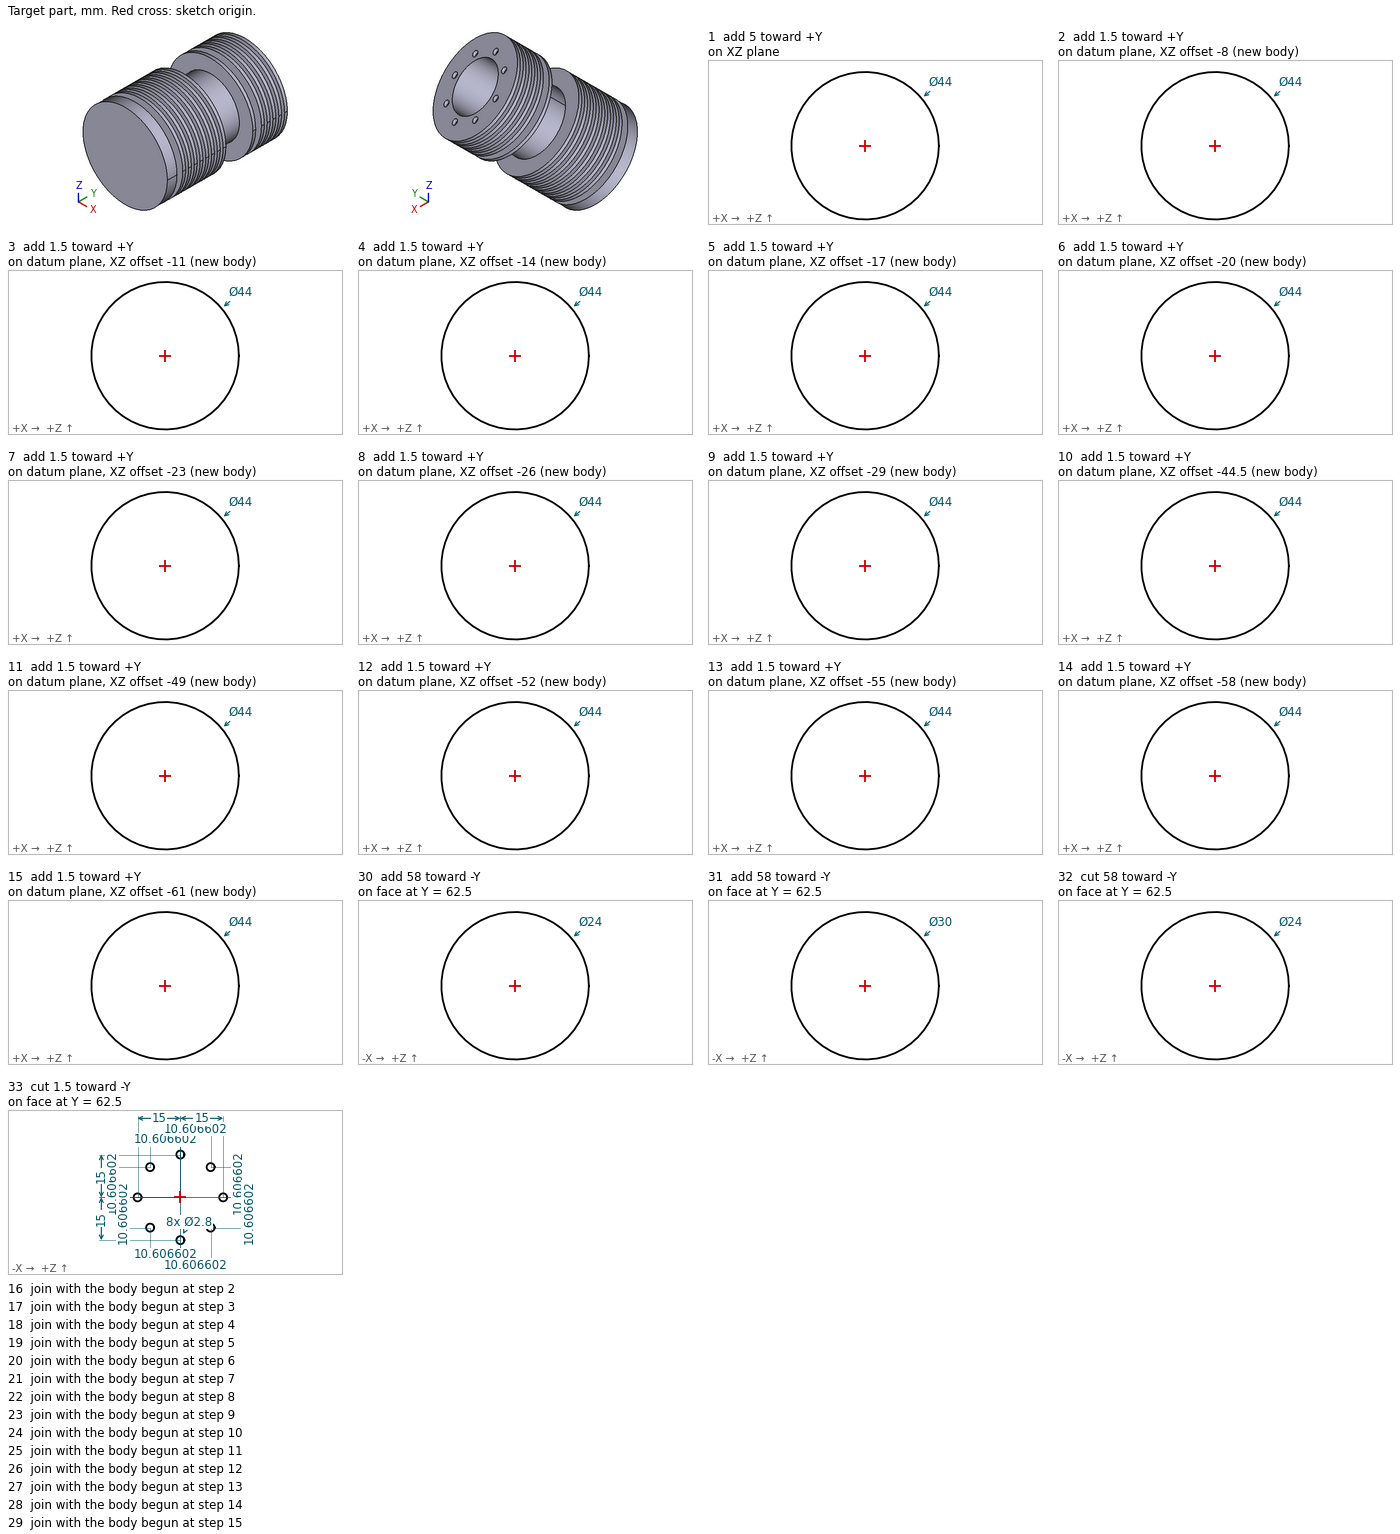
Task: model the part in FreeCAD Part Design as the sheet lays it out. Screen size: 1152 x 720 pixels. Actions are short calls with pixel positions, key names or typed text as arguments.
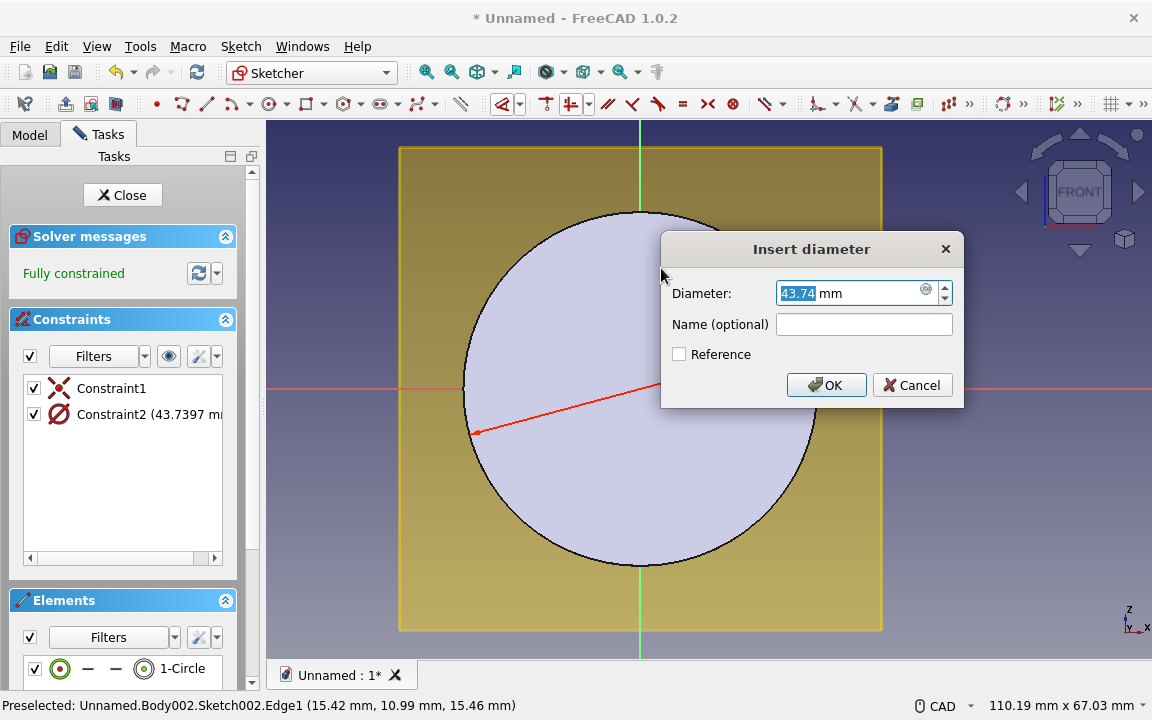
text(44)
key(Return)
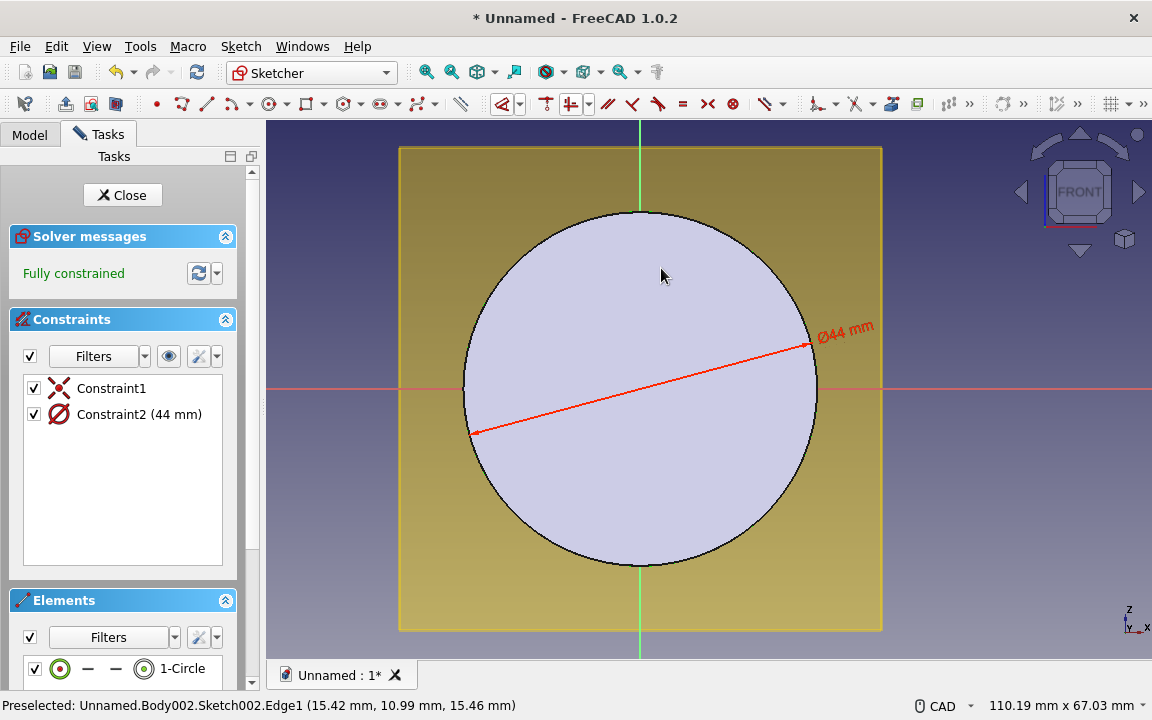
click(123, 195)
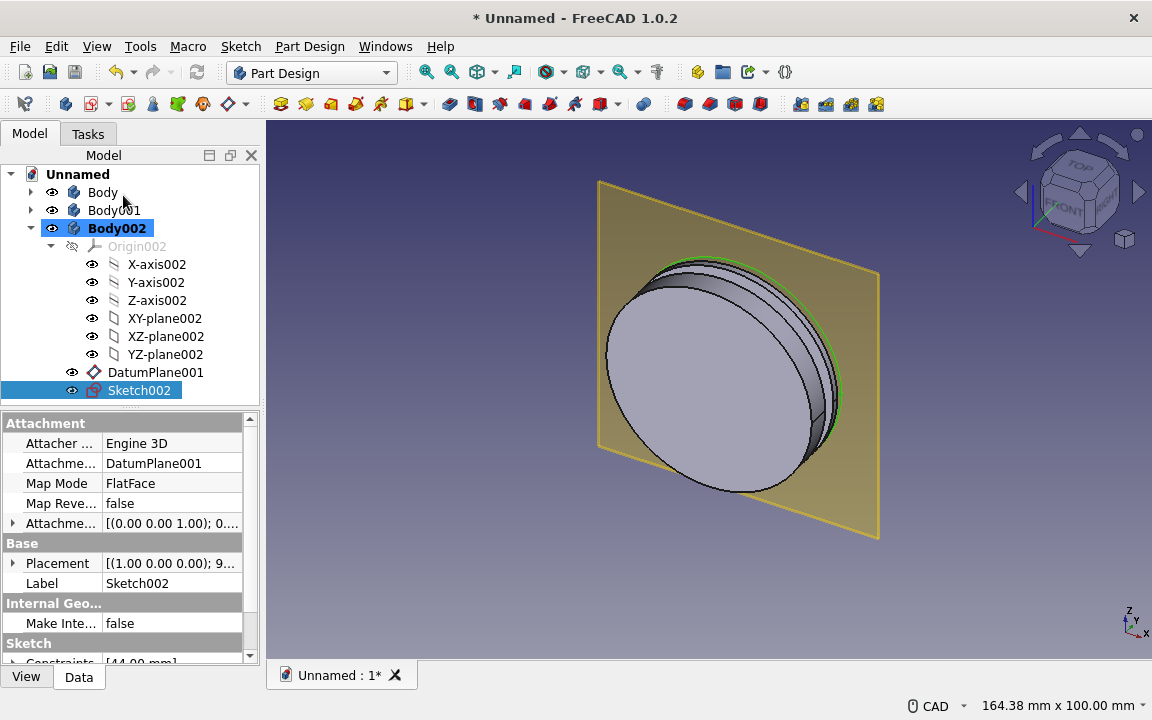
click(281, 104)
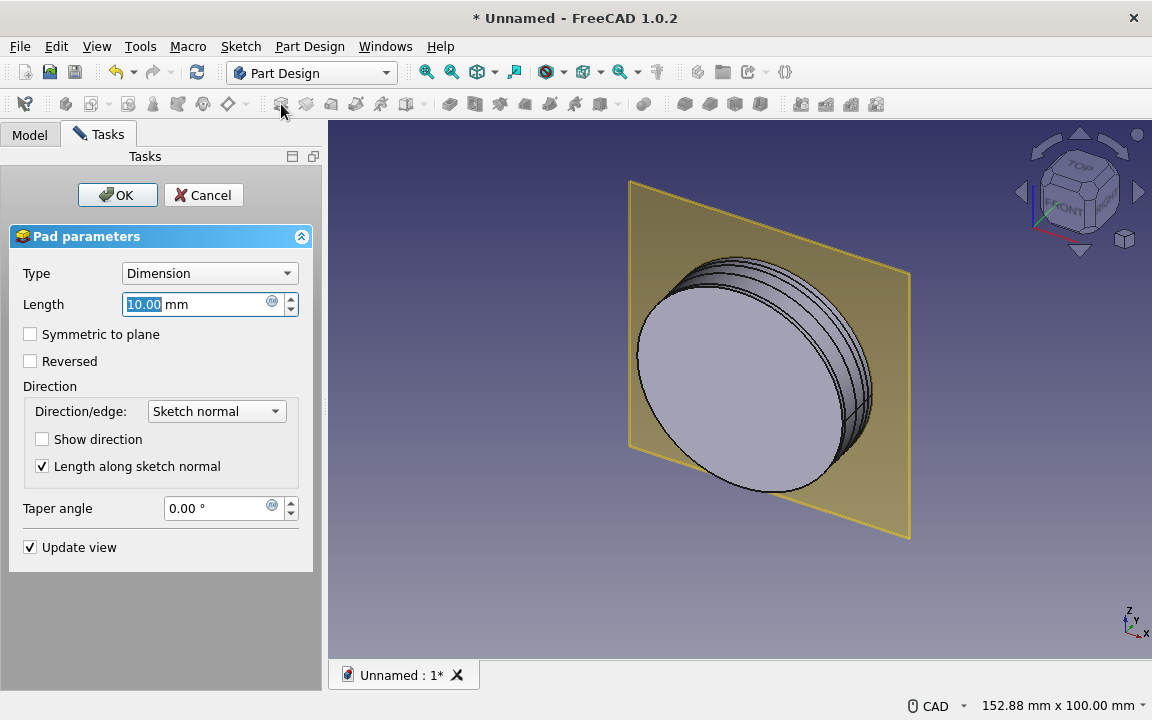
text(1.5)
key(Tab)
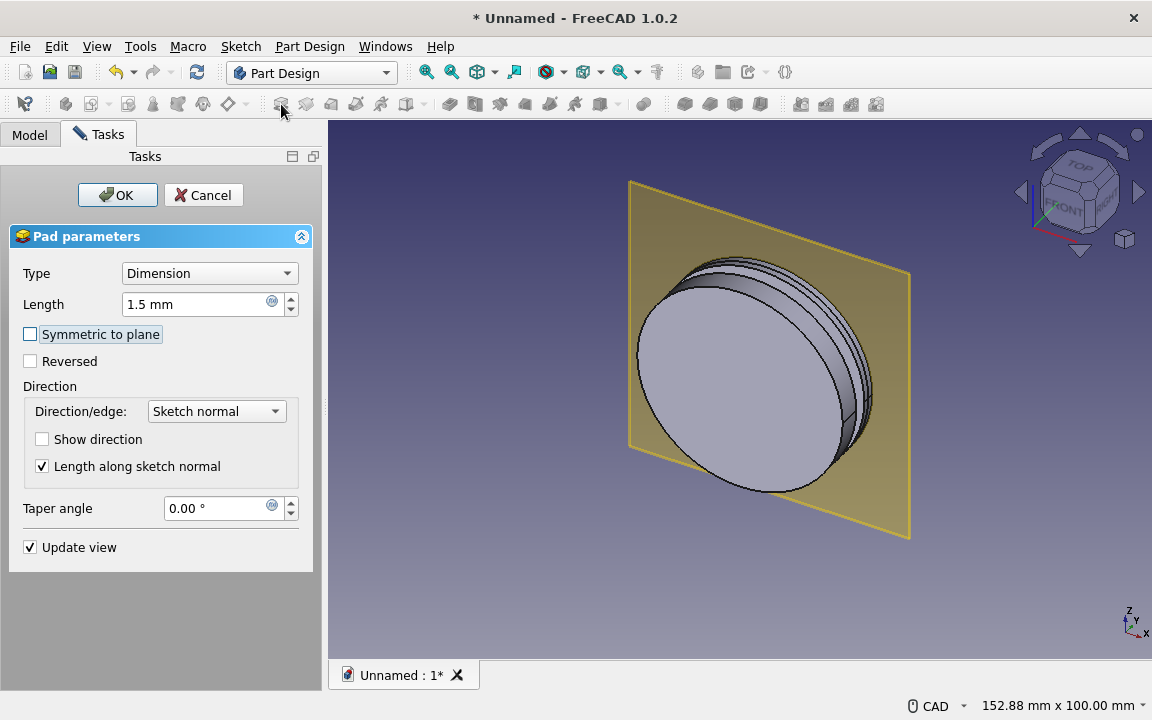
click(31, 361)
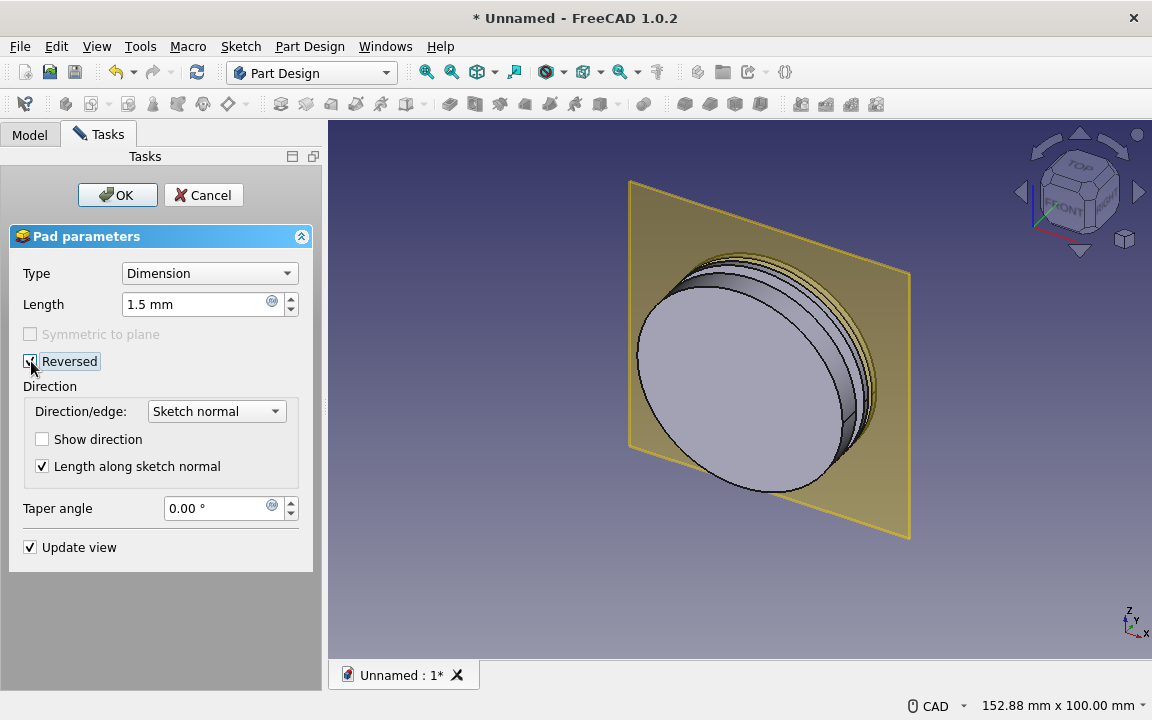
click(118, 195)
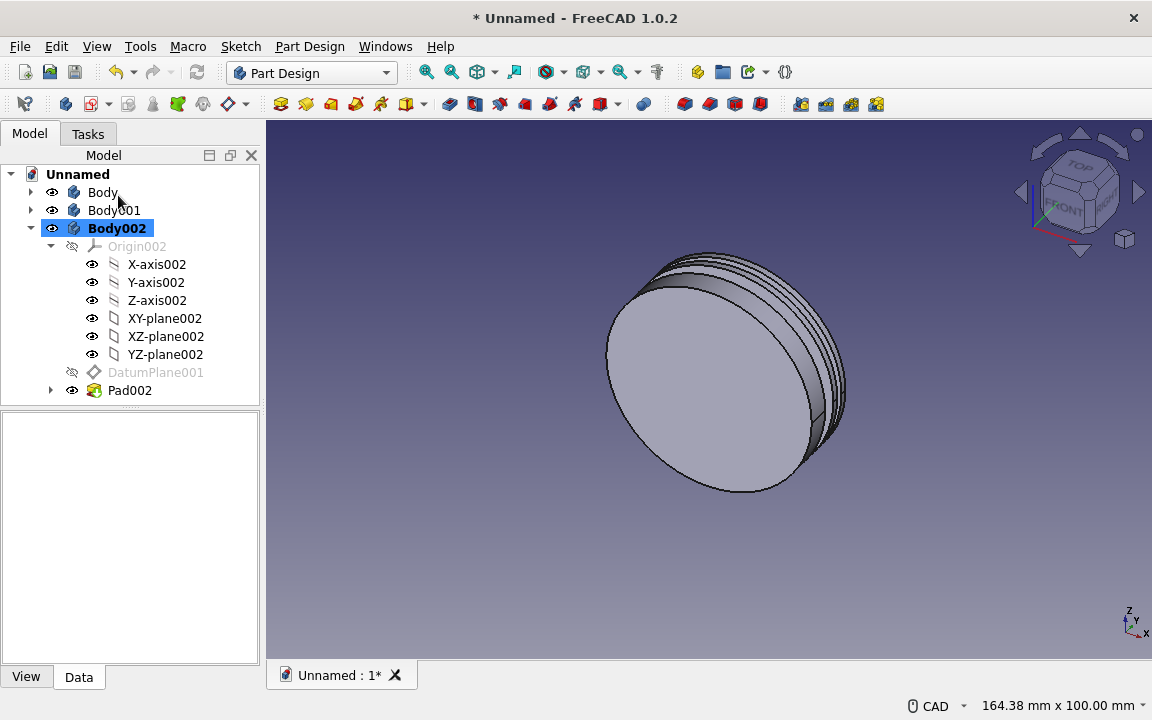
click(66, 104)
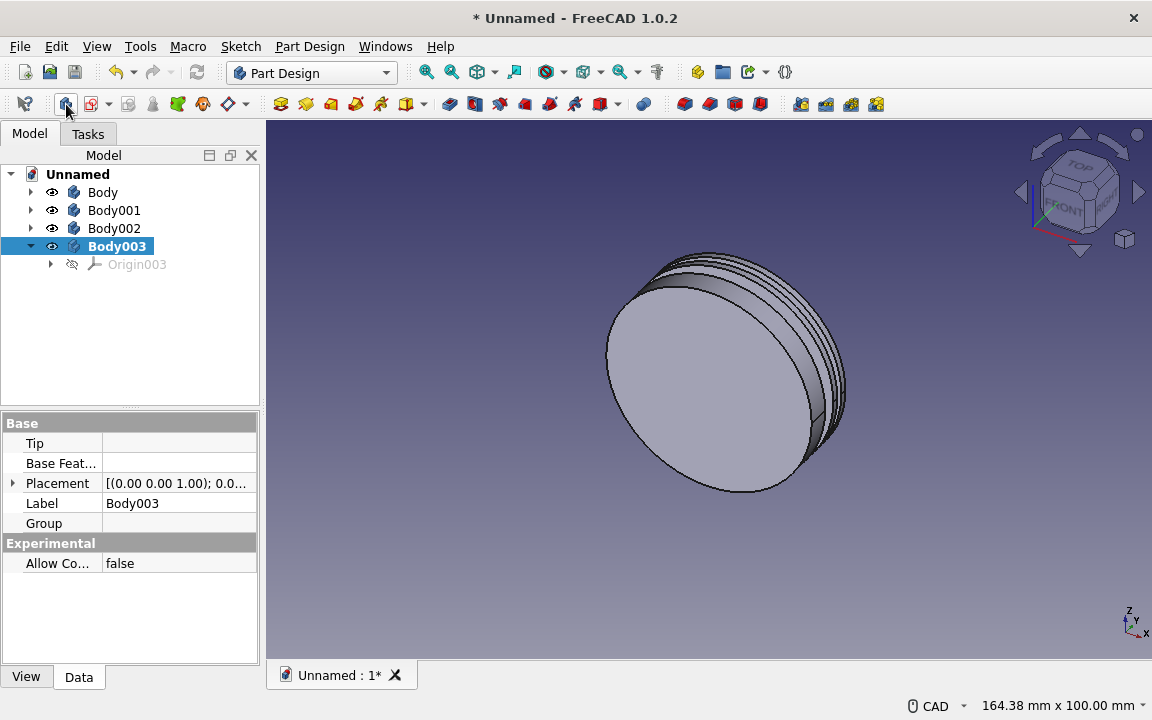
click(51, 264)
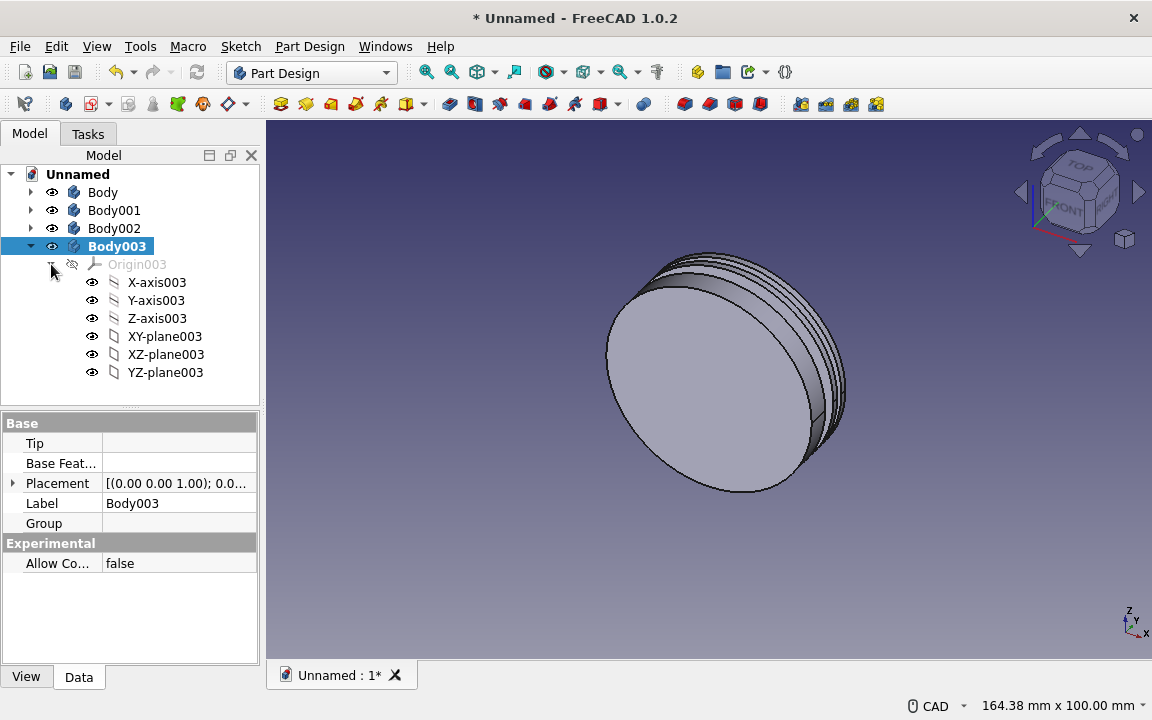
click(137, 354)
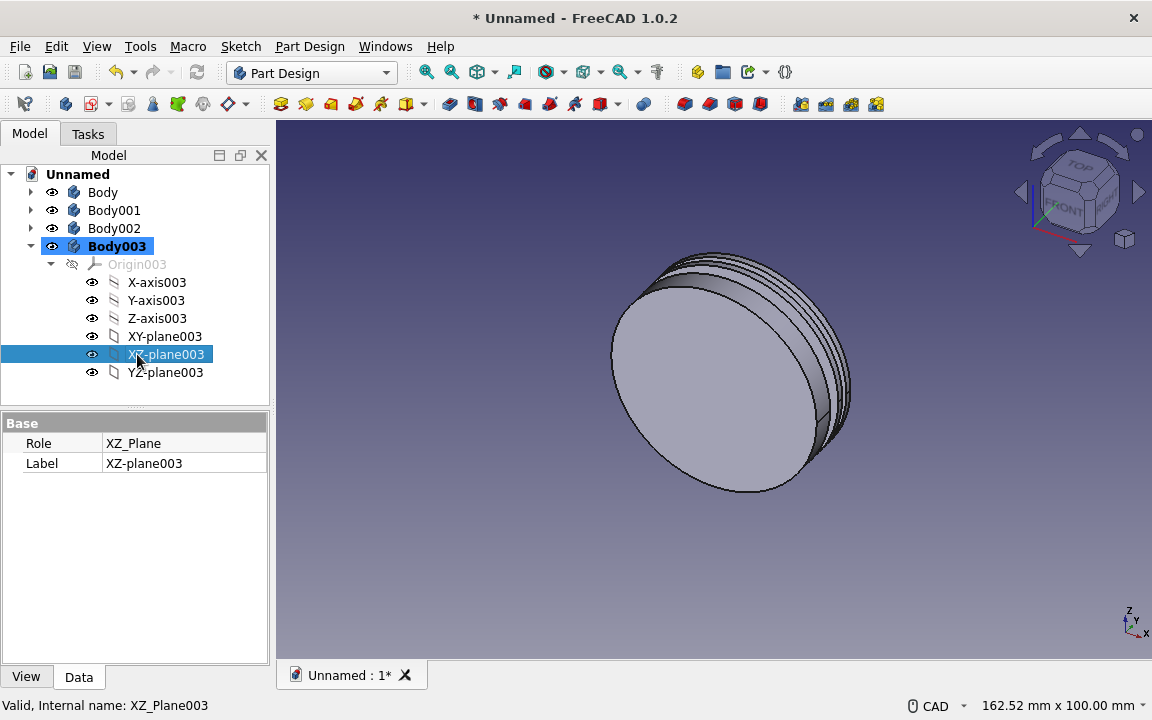
click(228, 104)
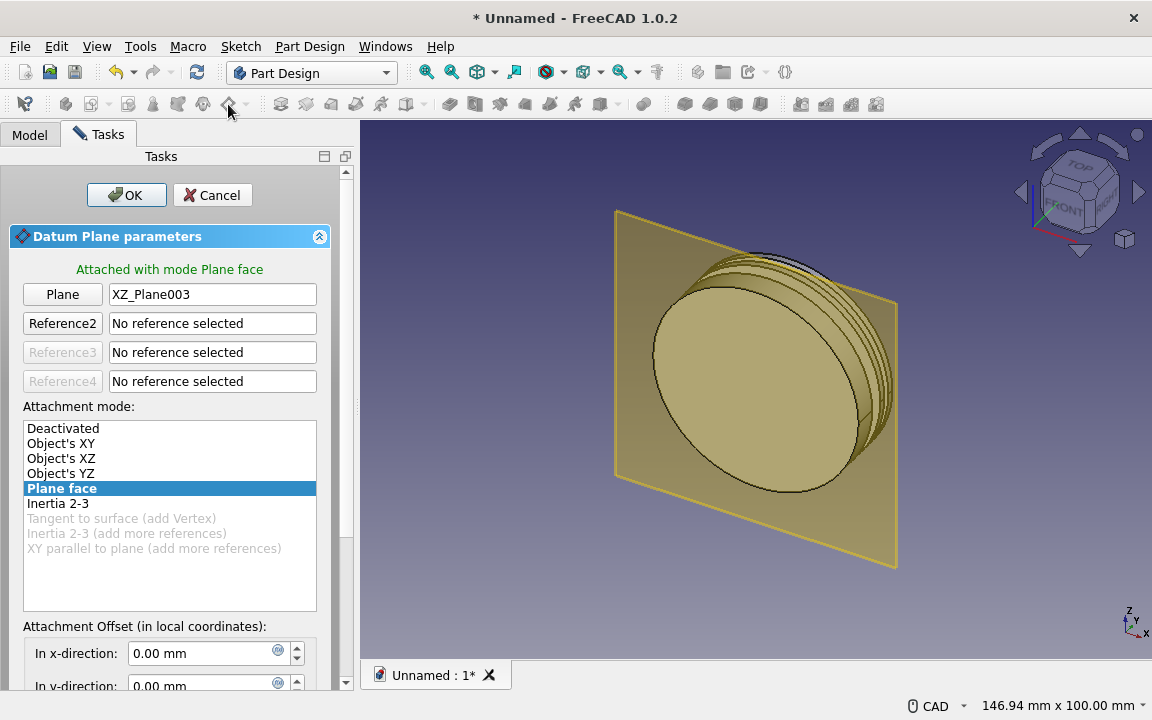
scroll(346, 428, down, 2)